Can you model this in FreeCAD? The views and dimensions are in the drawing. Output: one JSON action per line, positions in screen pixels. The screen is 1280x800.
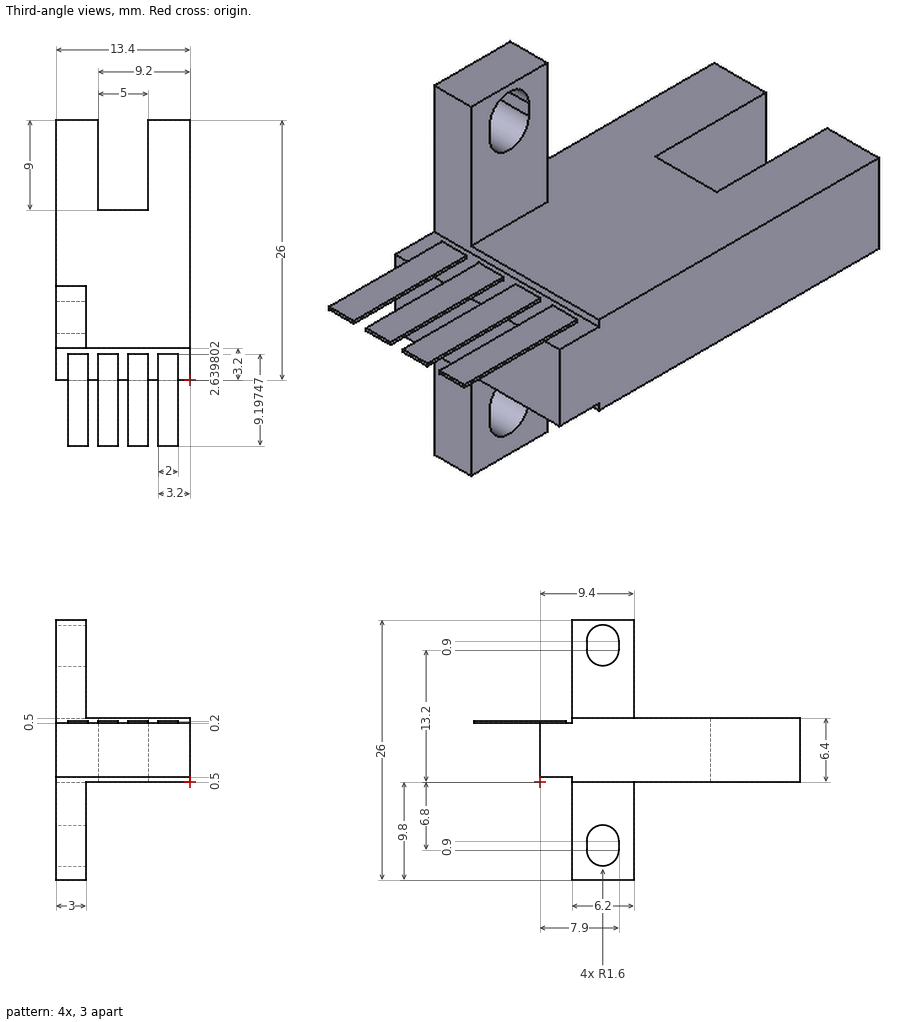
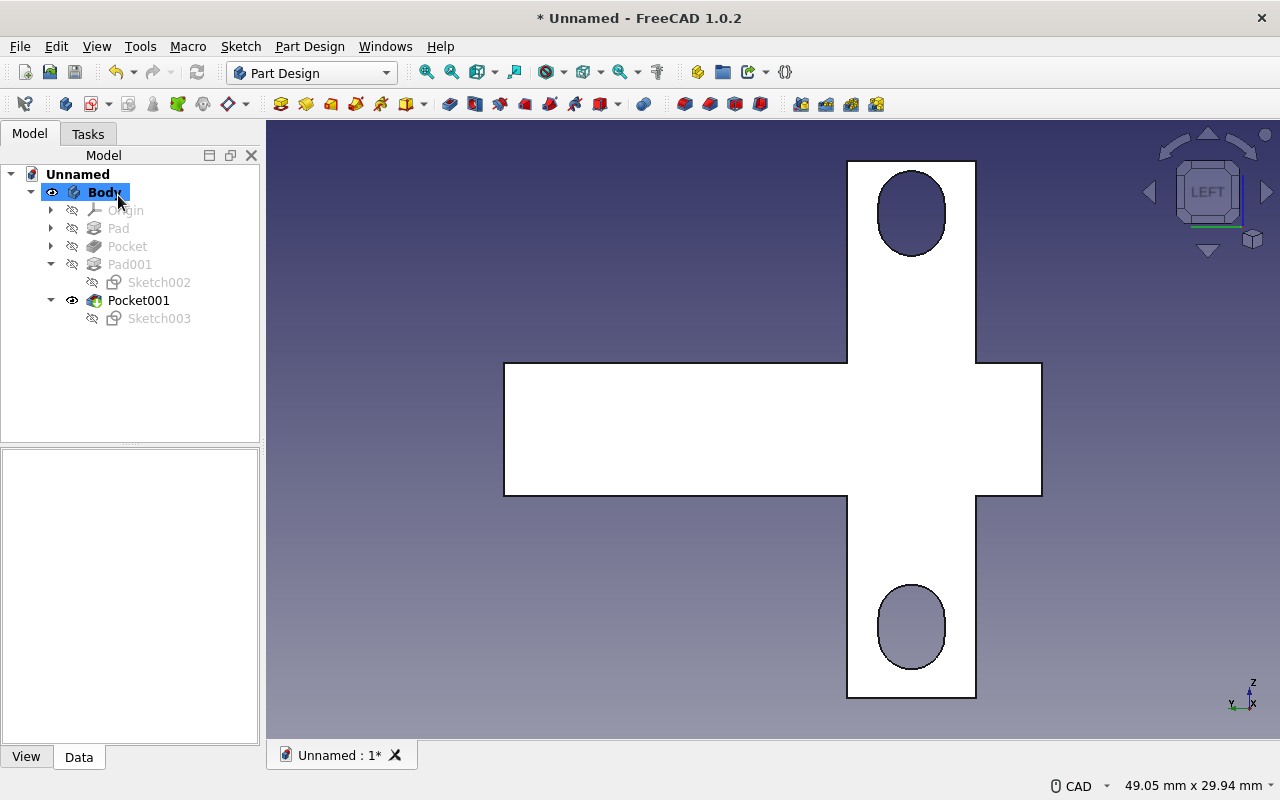
{"action": "key", "text": "0"}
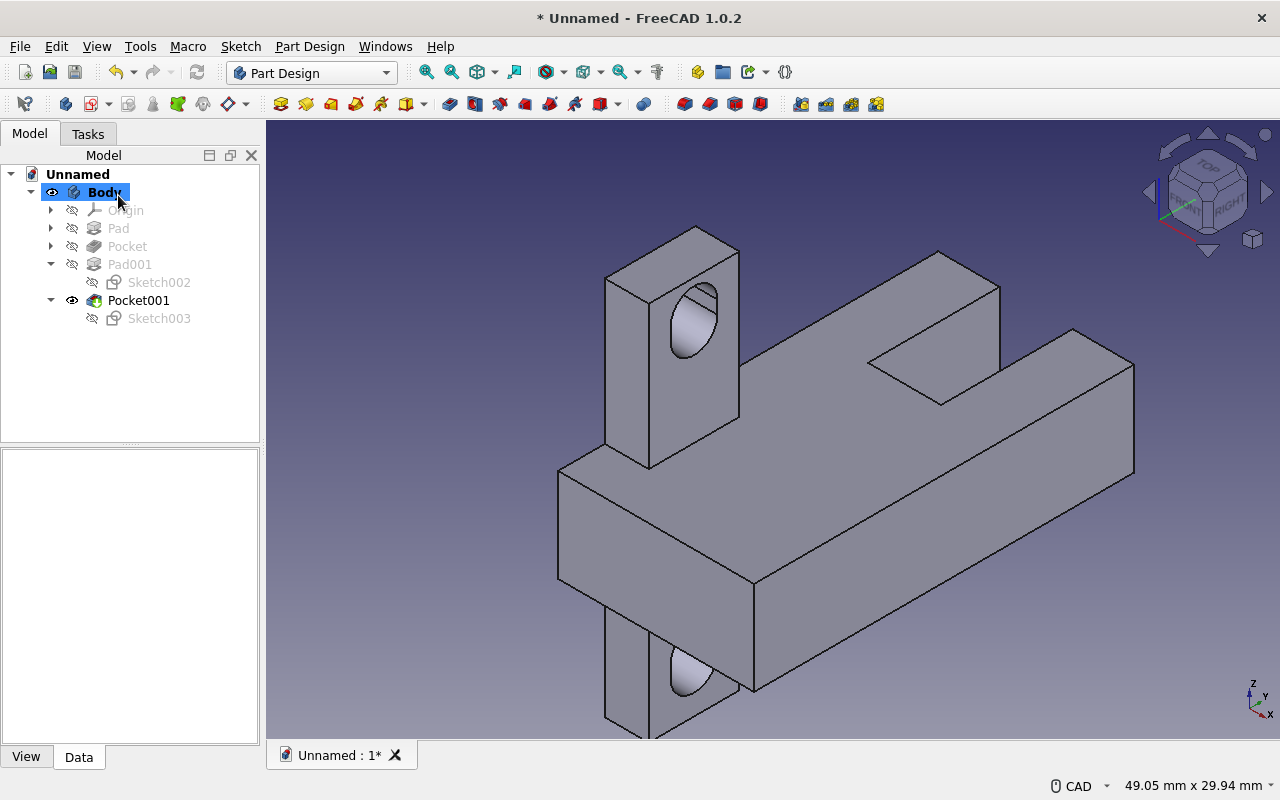
{"action": "left_click", "coordinate": [427, 72]}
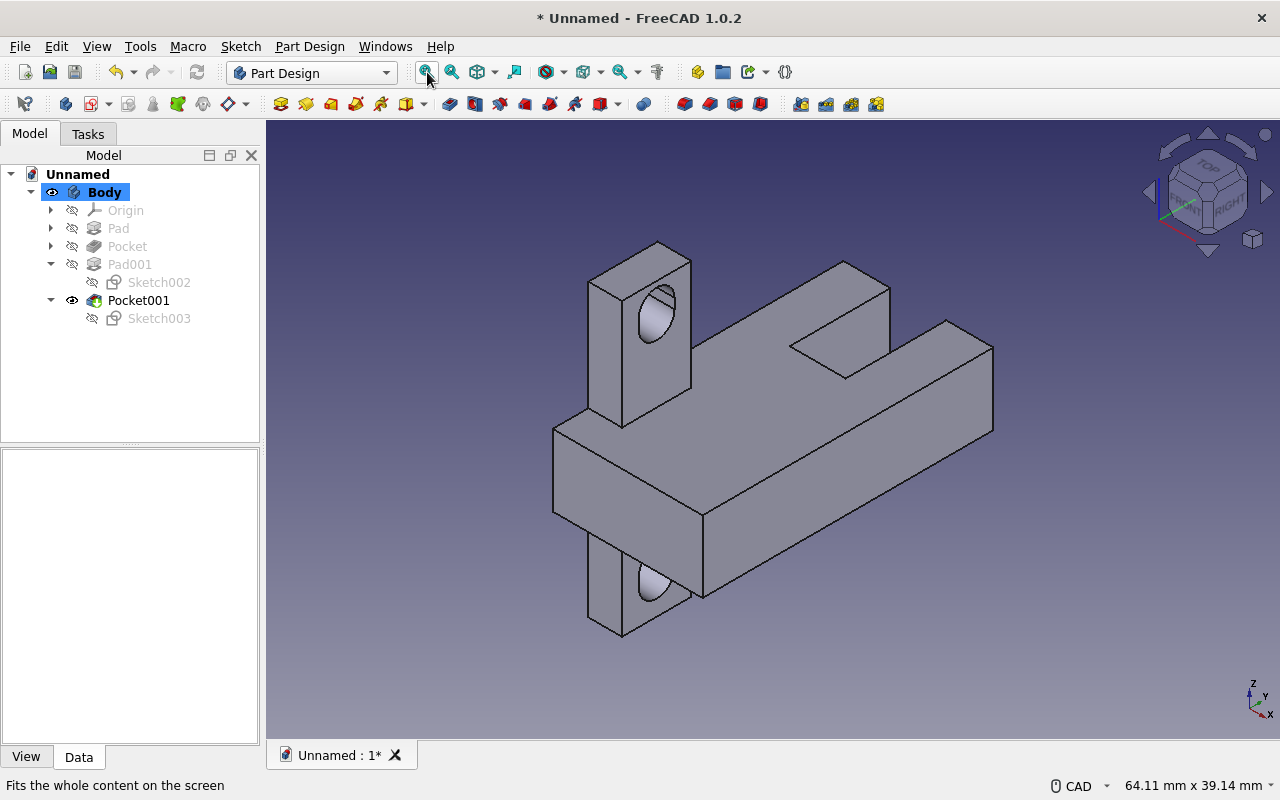
{"action": "left_click", "coordinate": [753, 424]}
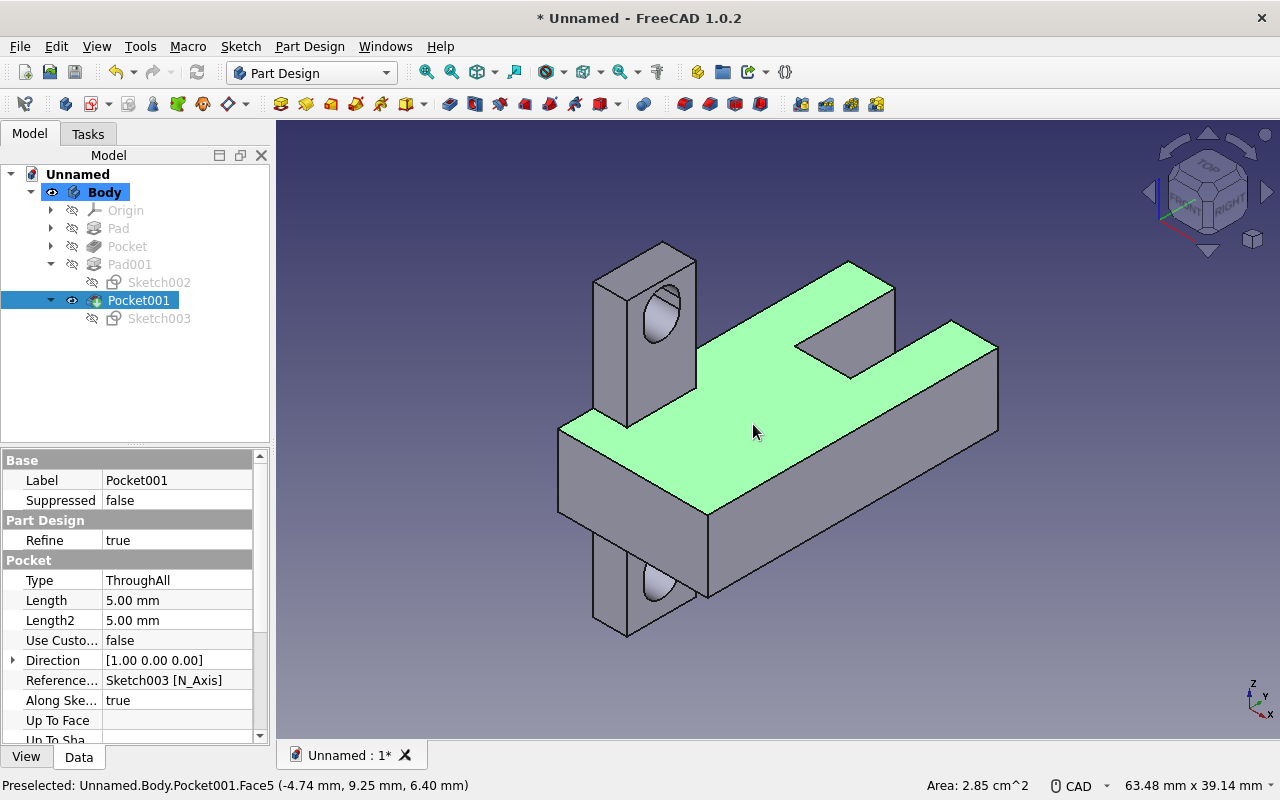
{"action": "left_click", "coordinate": [90, 104]}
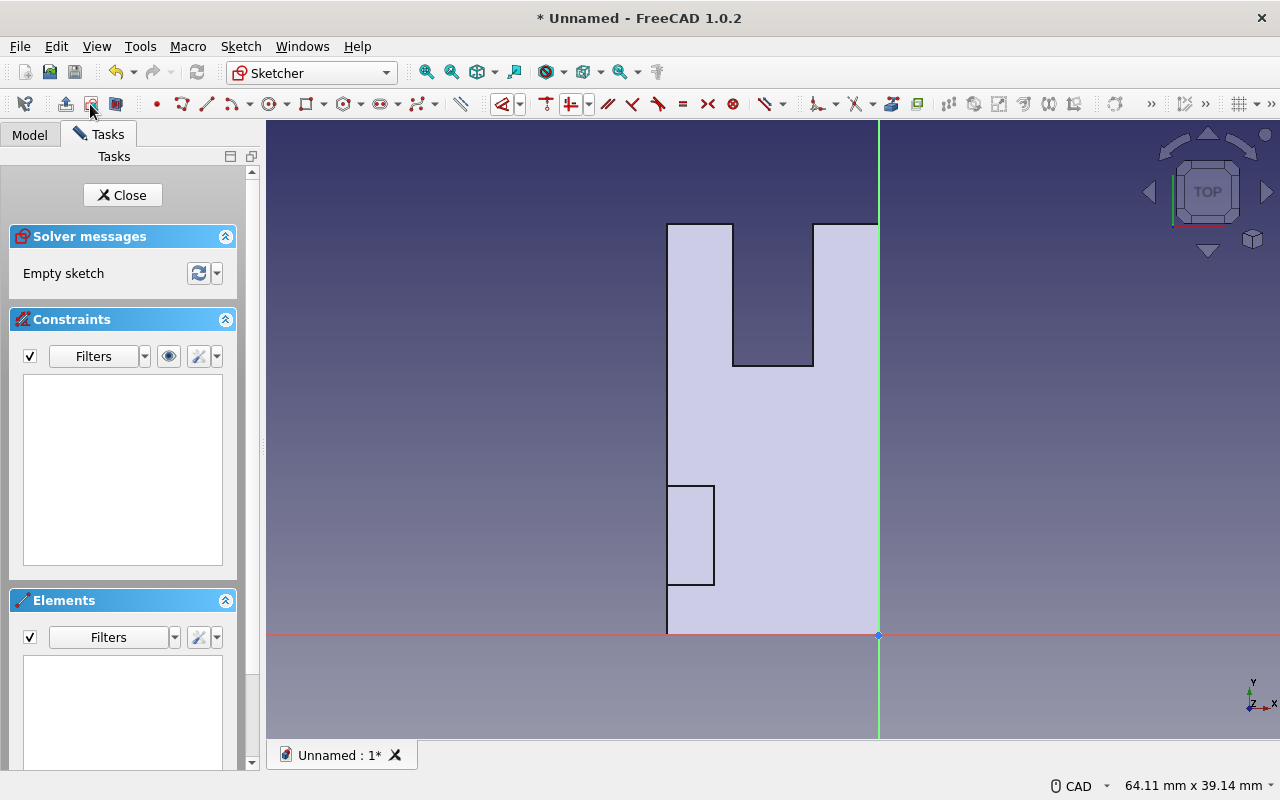
{"action": "scroll", "coordinate": [813, 711], "scroll_direction": "up", "scroll_amount": 5}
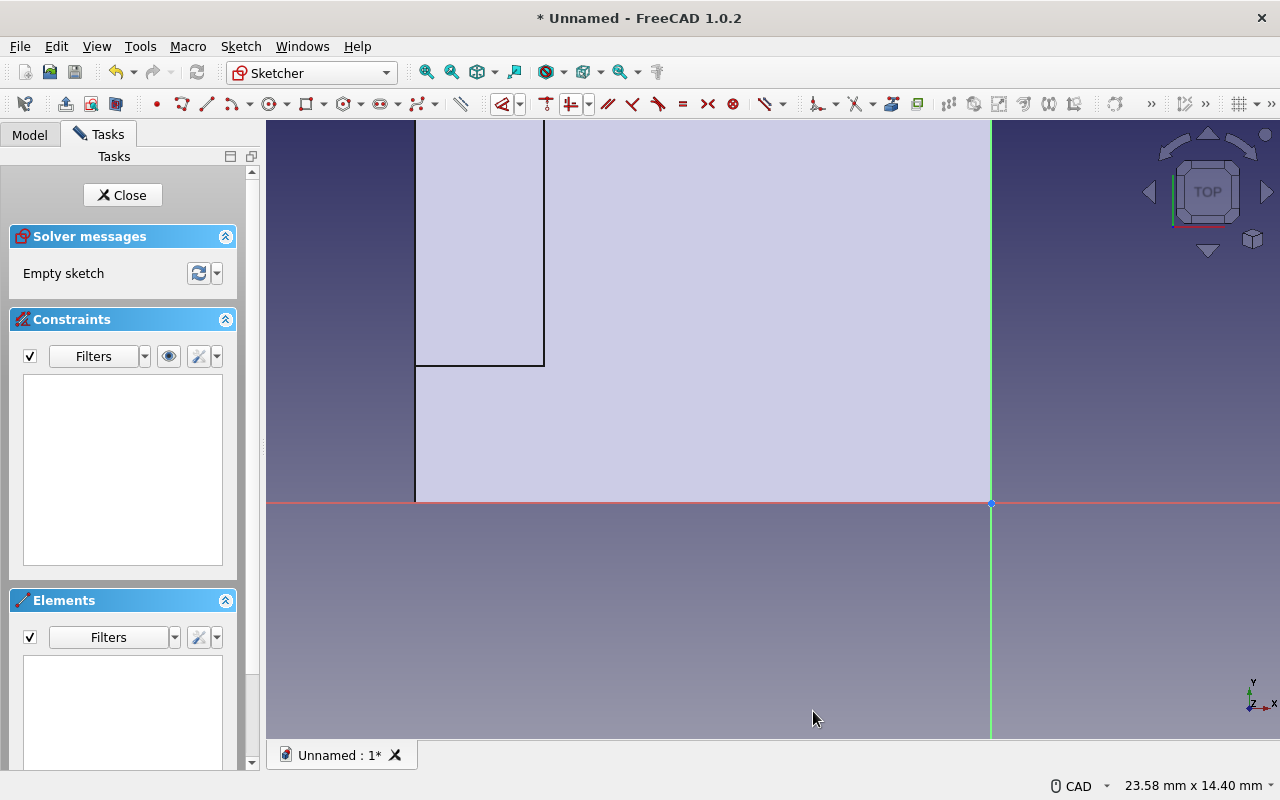
{"action": "left_click", "coordinate": [306, 104]}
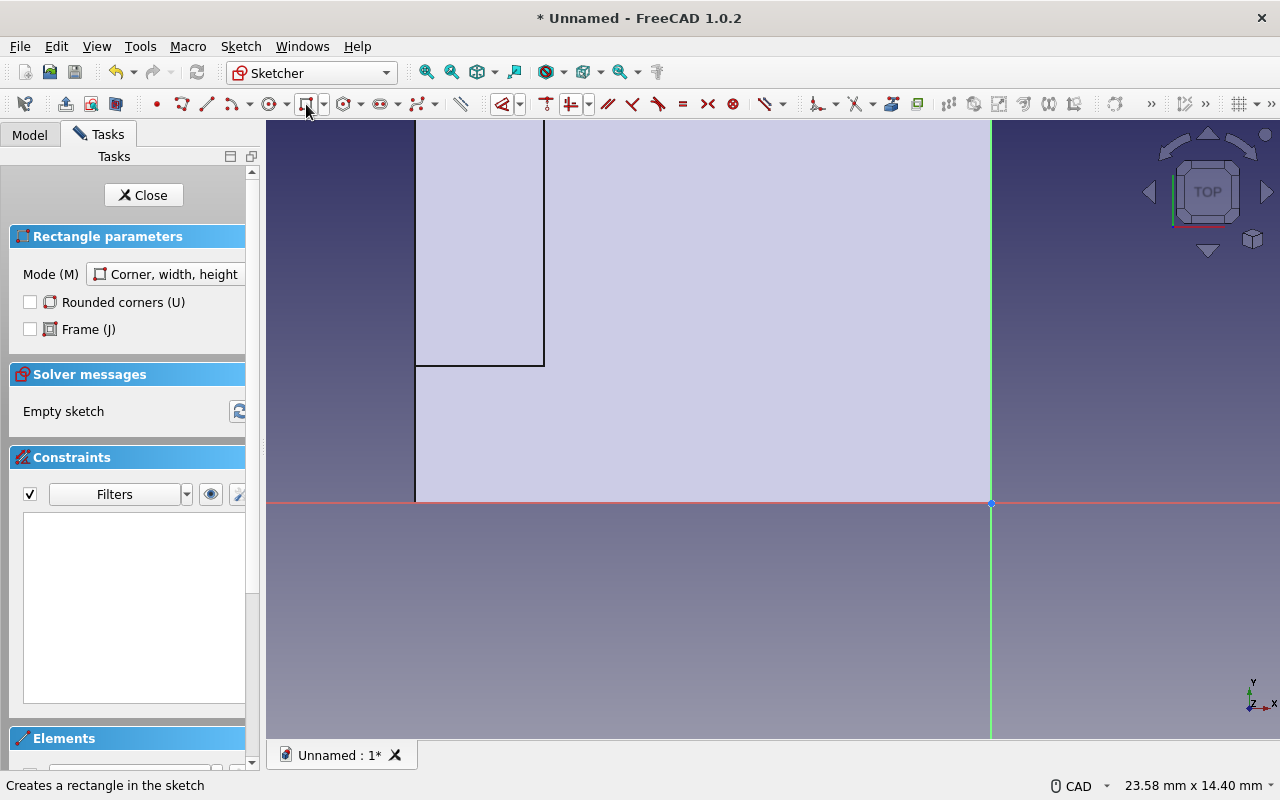
{"action": "left_click", "coordinate": [991, 503]}
{"action": "left_click", "coordinate": [415, 366]}
{"action": "key", "text": "Escape"}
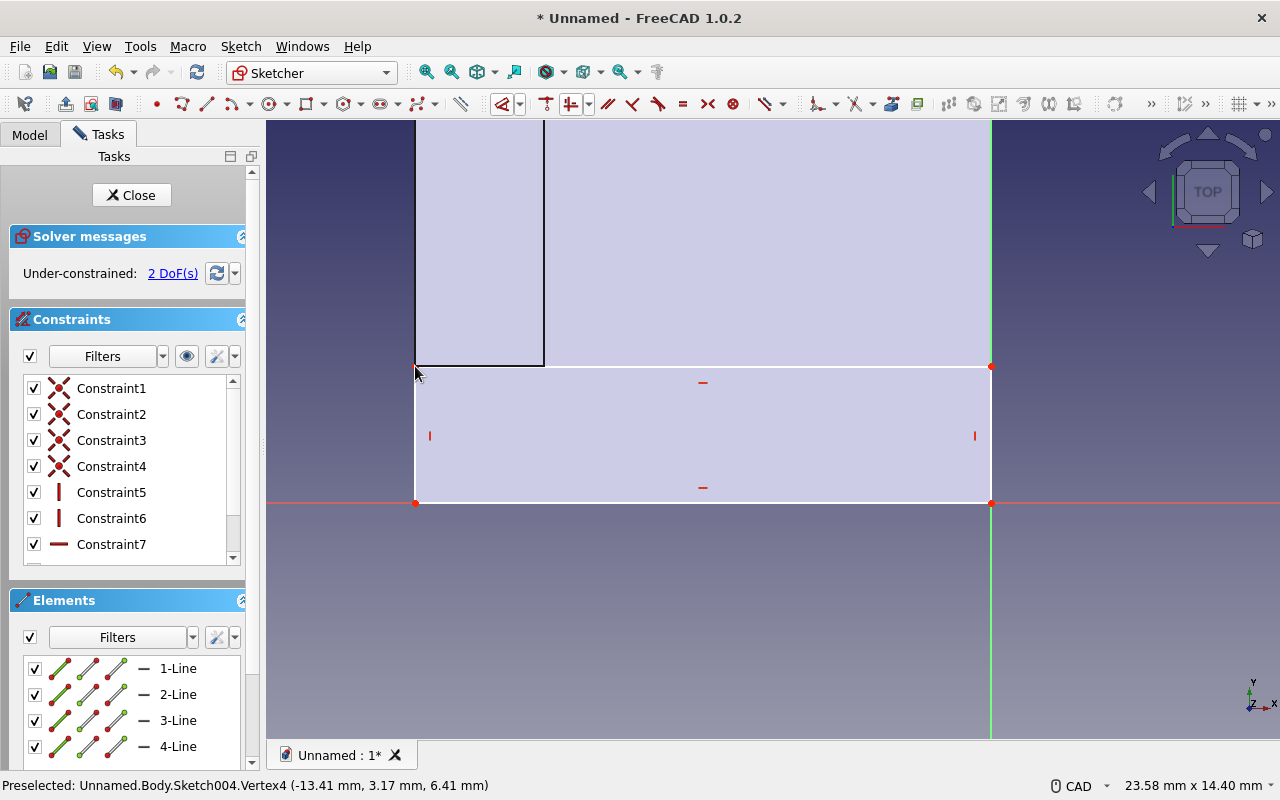
{"action": "left_click", "coordinate": [991, 462]}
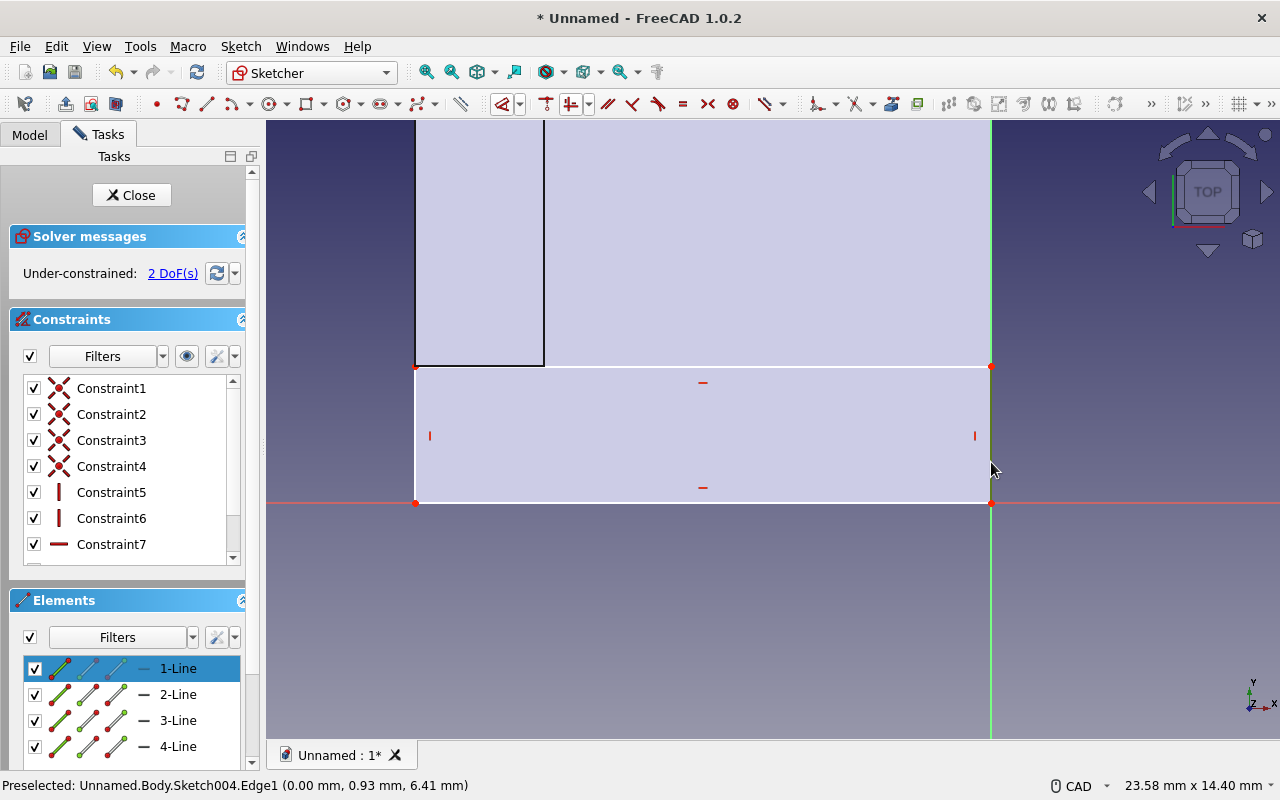
{"action": "key", "text": "i"}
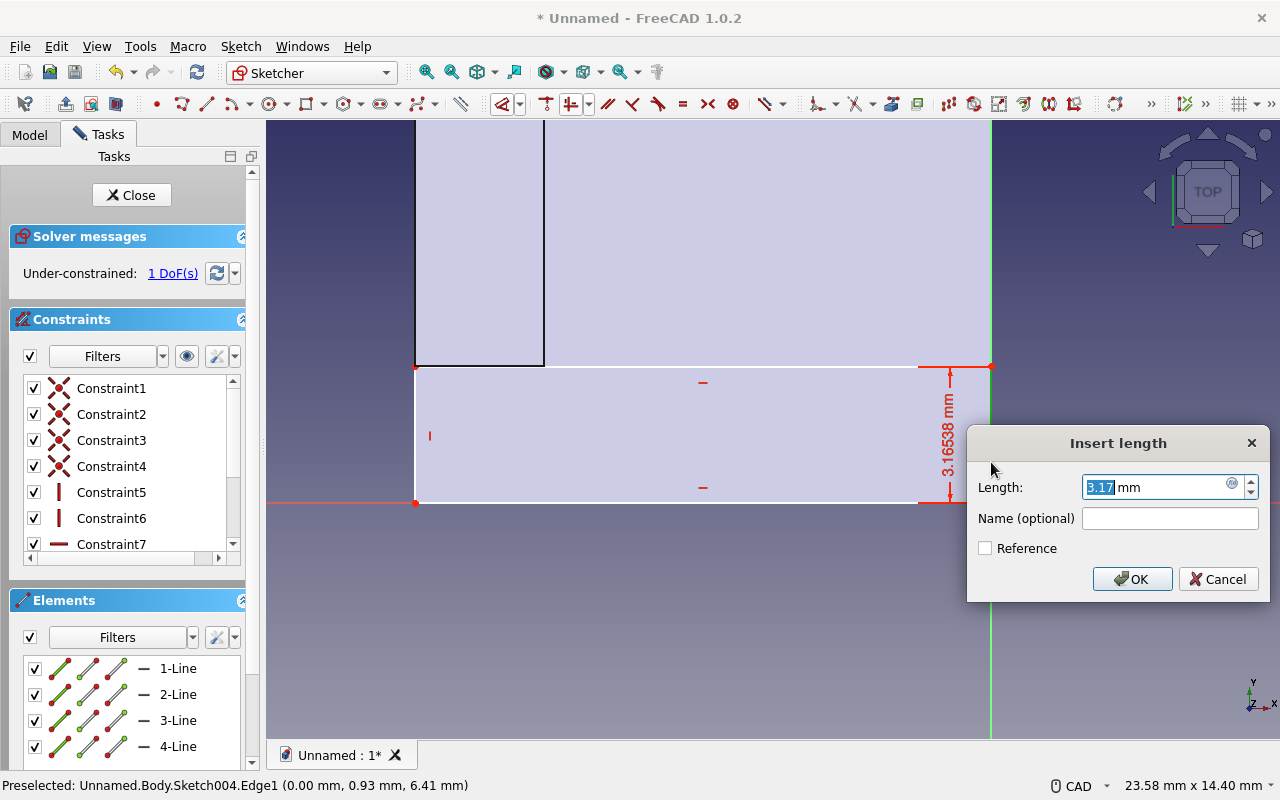
{"action": "type", "text": "3.2"}
{"action": "key", "text": "Return"}